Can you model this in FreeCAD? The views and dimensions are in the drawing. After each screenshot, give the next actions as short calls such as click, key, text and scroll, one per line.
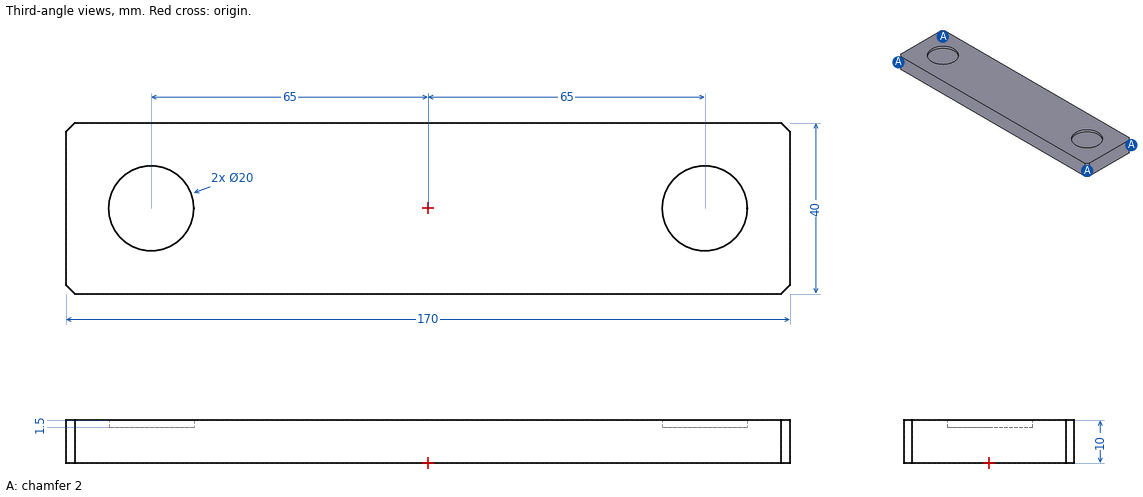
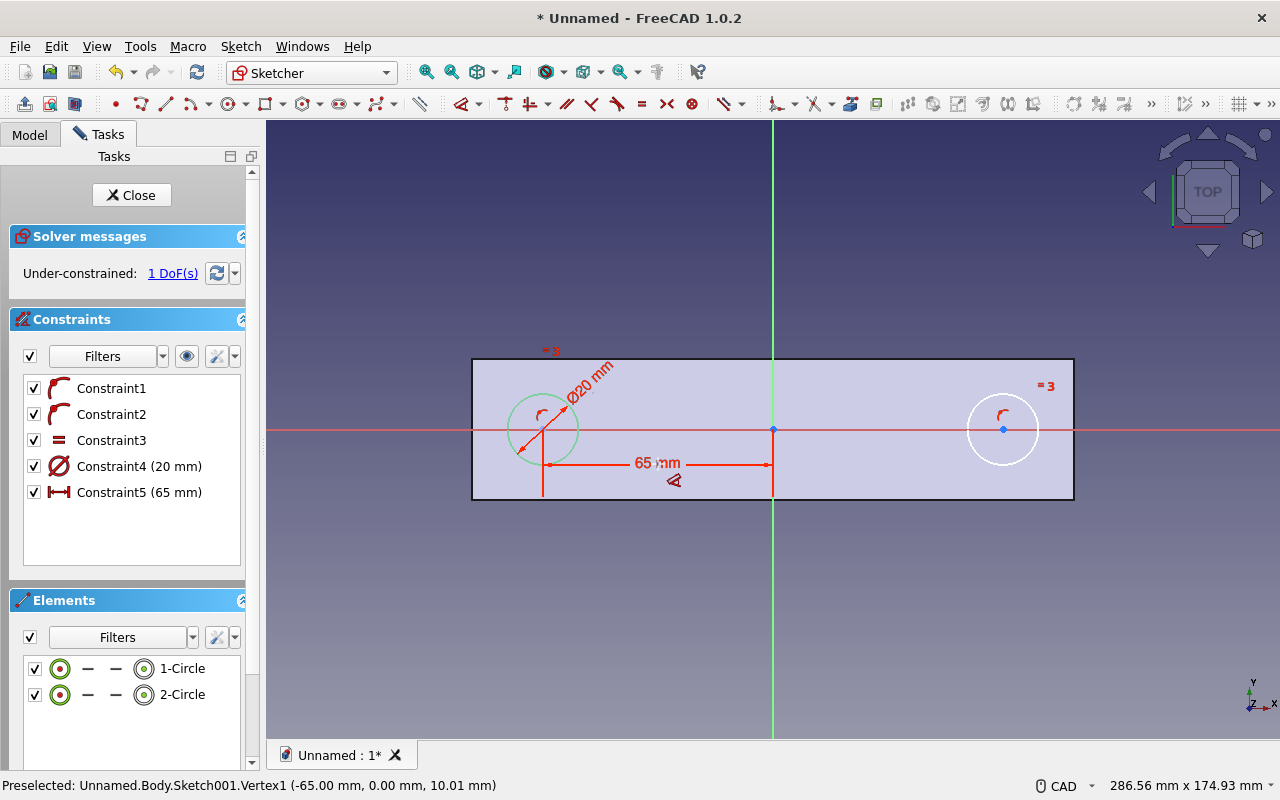
click(1003, 430)
click(888, 464)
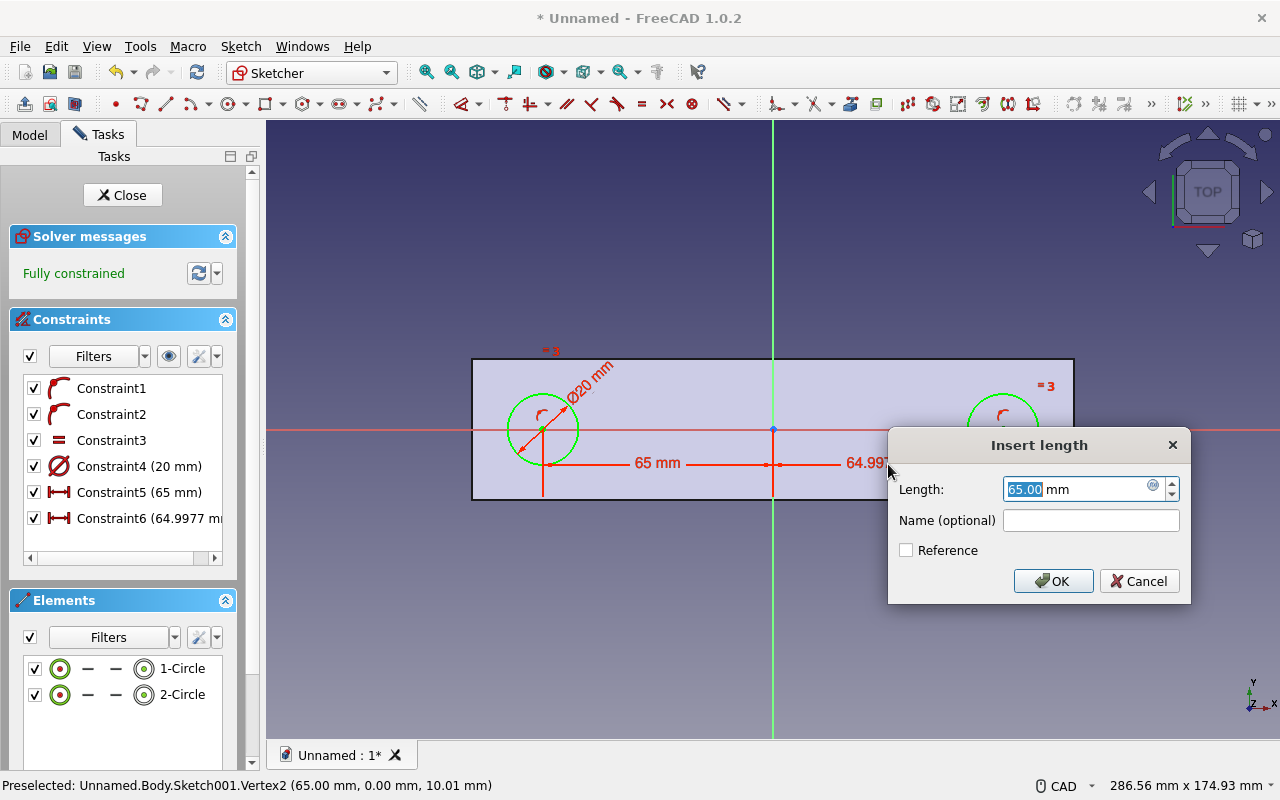
text(65)
key(Return)
key(Escape)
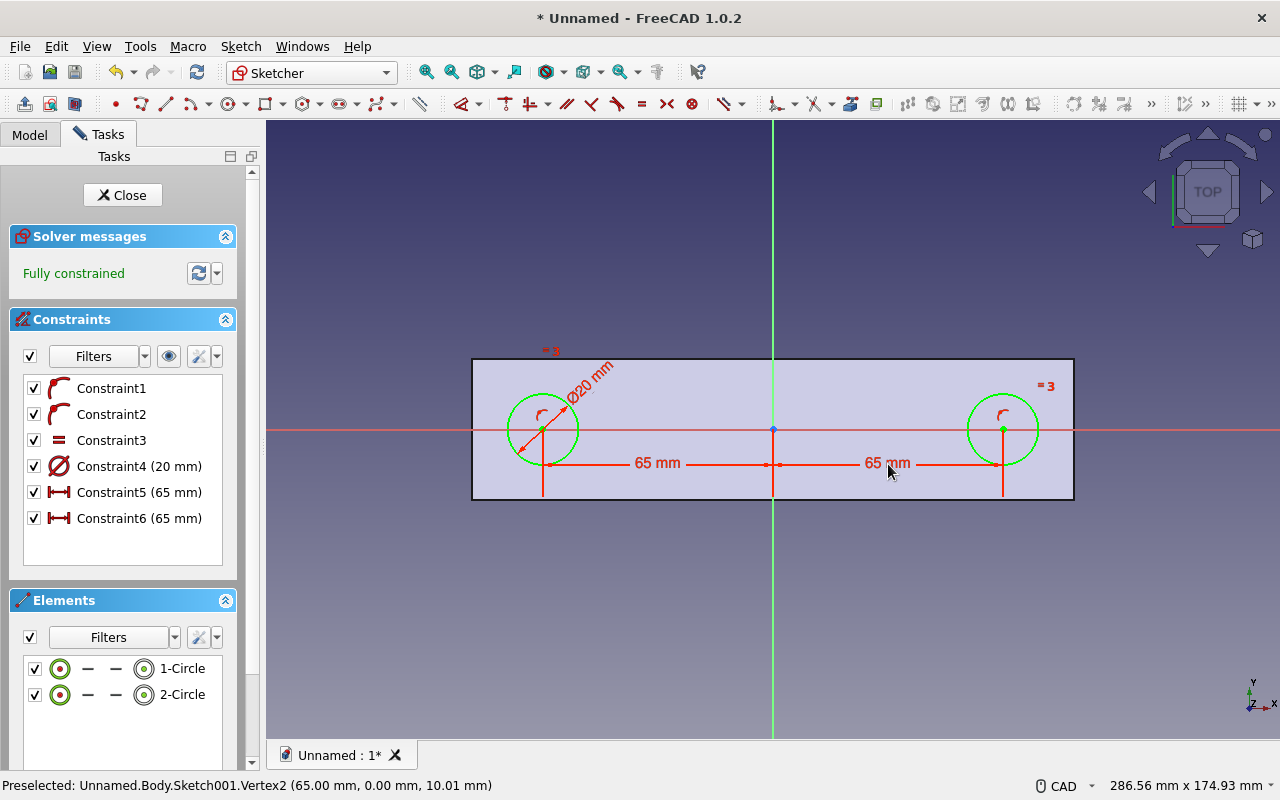
click(123, 195)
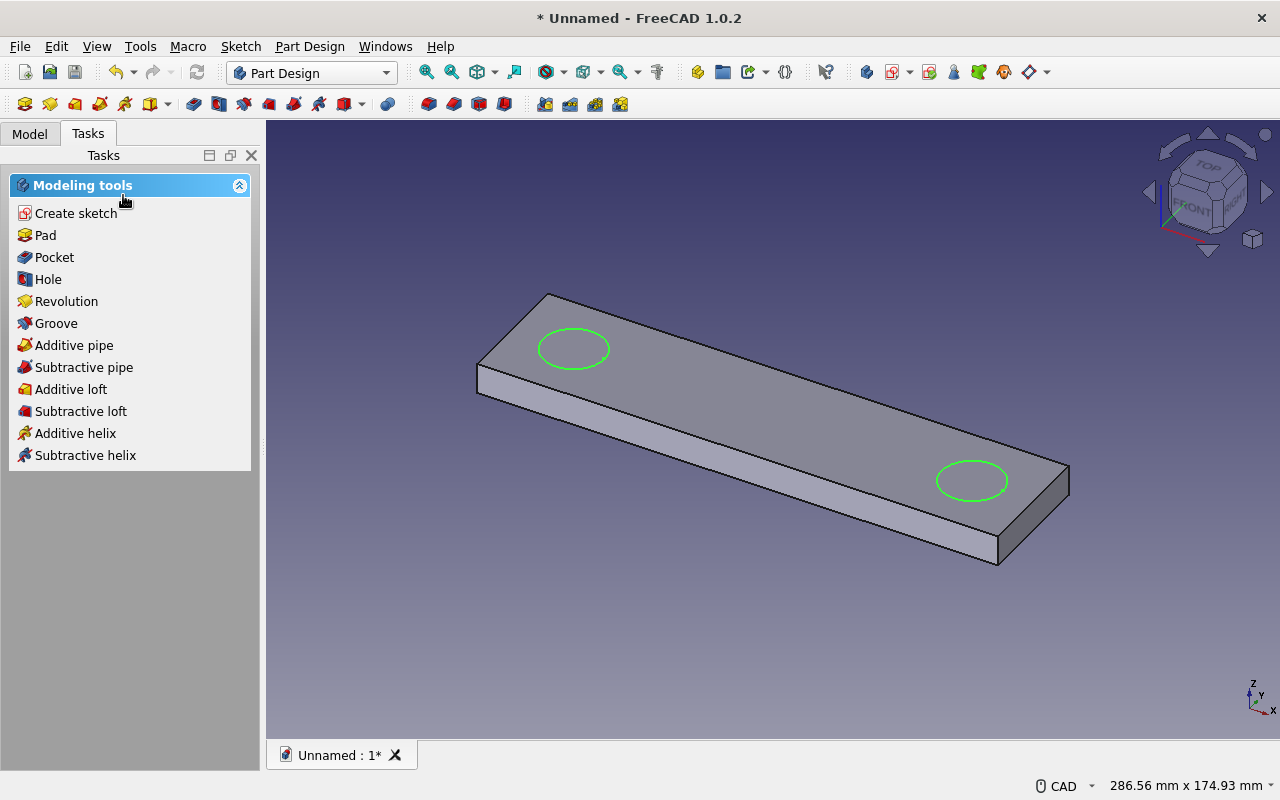
click(194, 104)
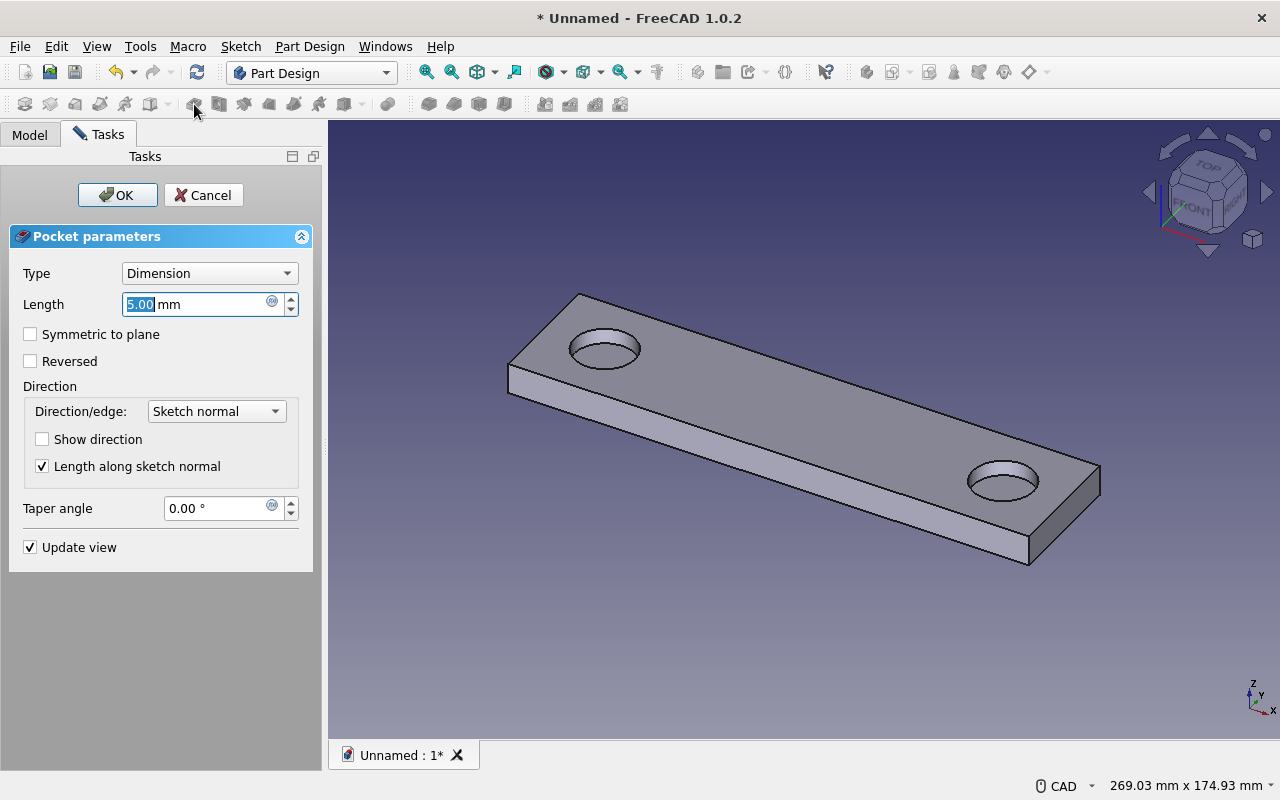
text(1.5)
key(Tab)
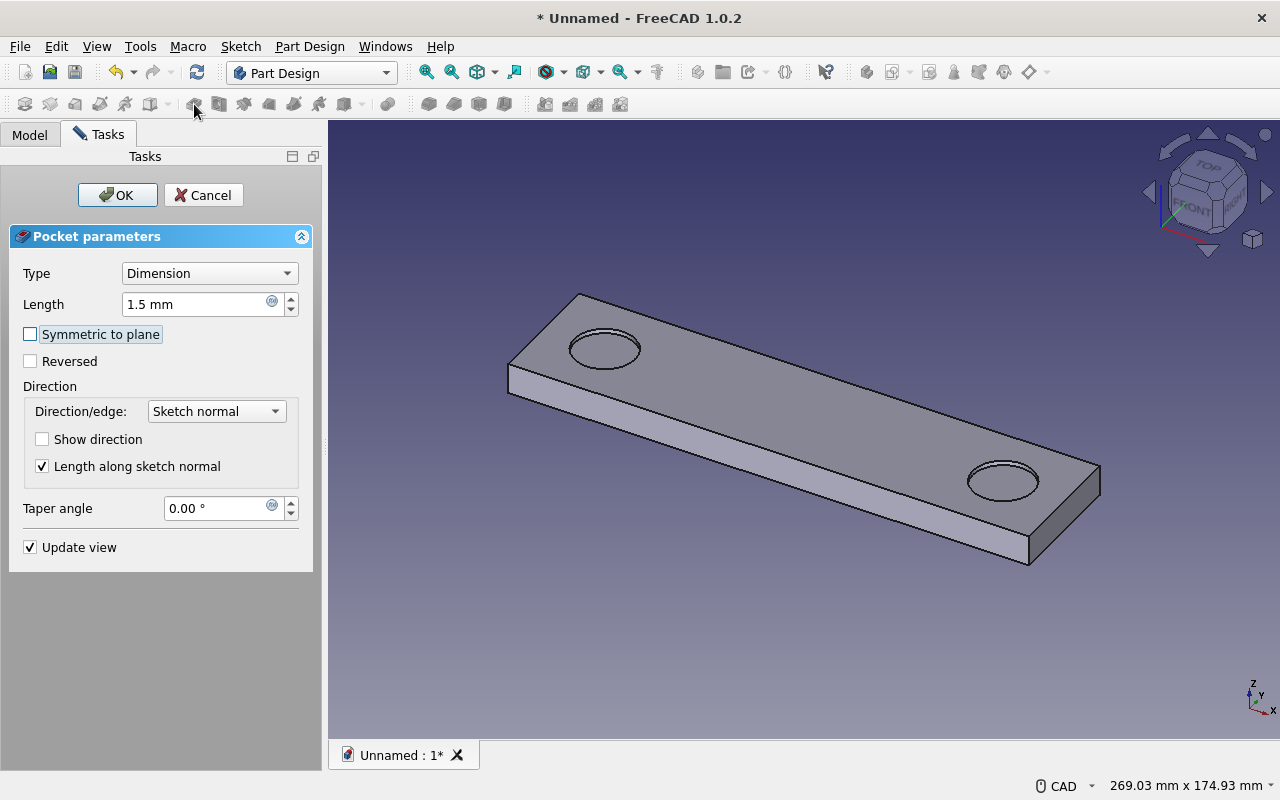
click(118, 195)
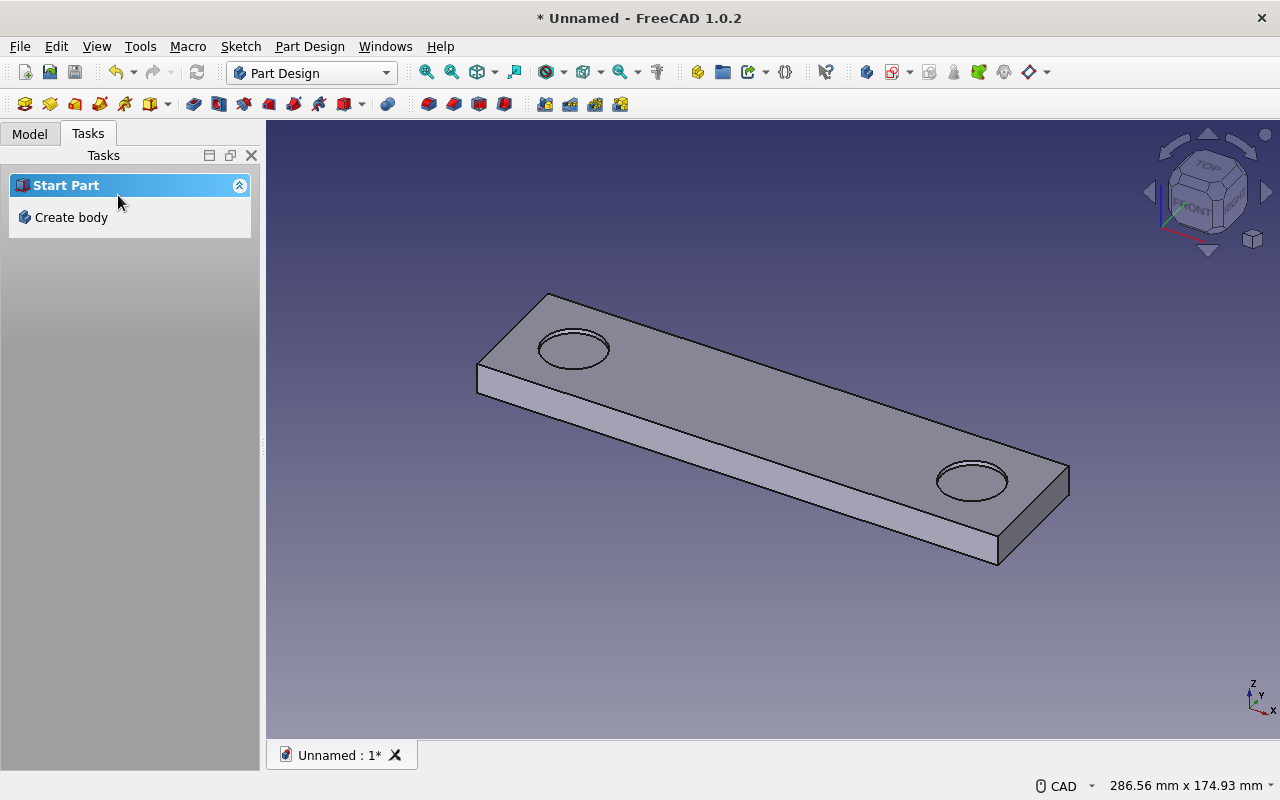
click(998, 550)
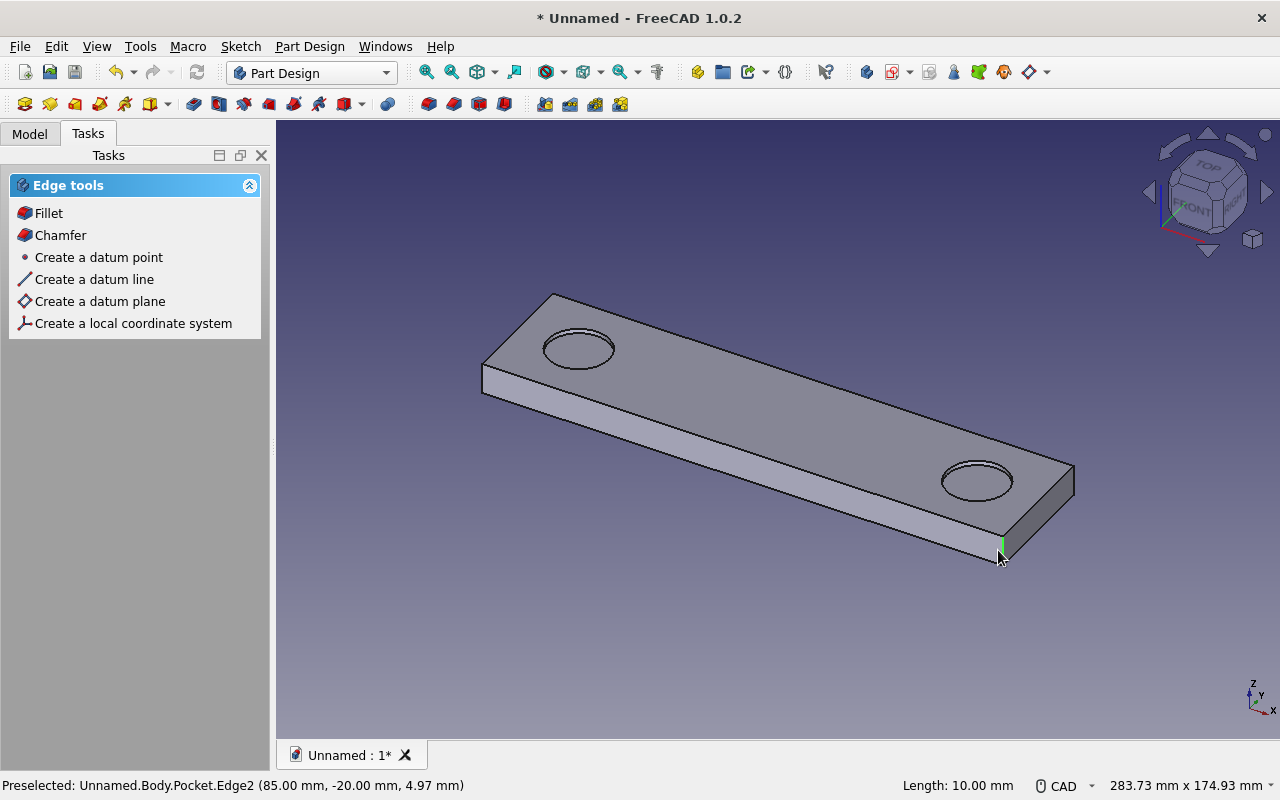
key(0)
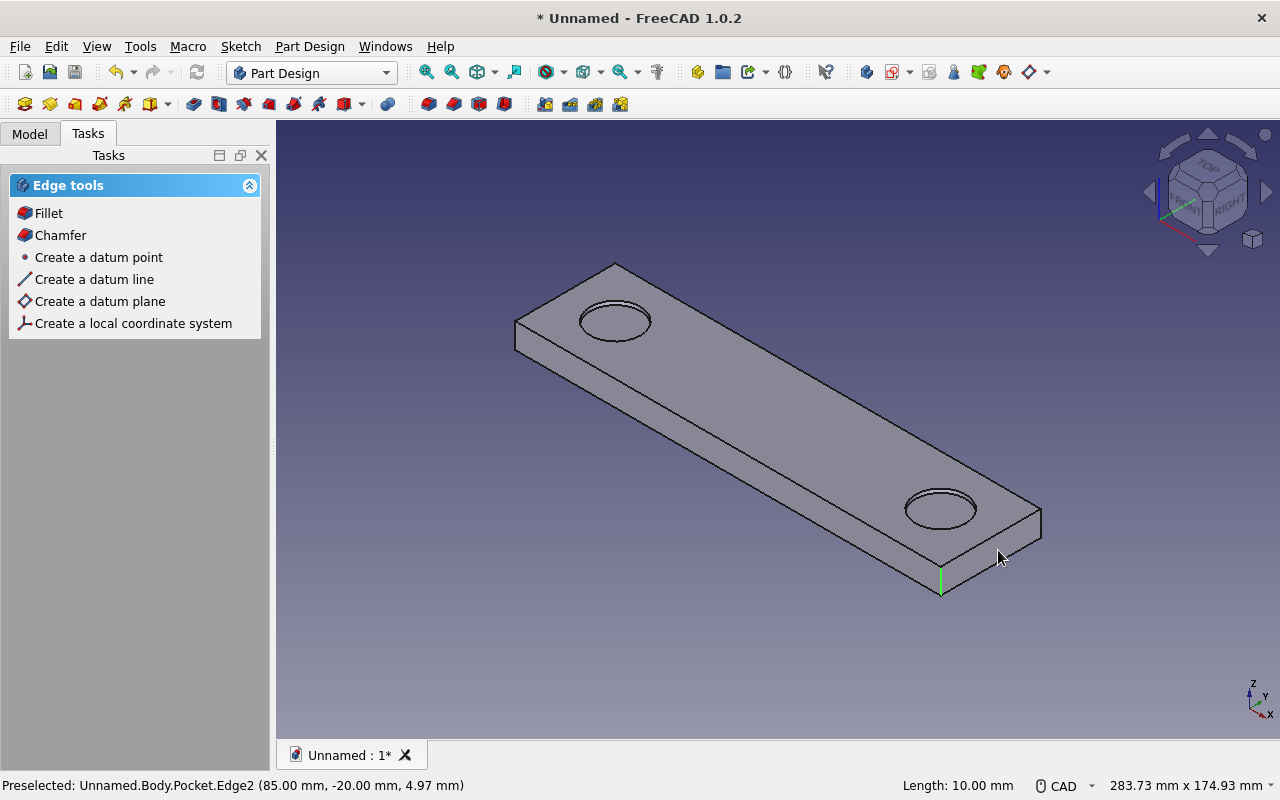
key(2)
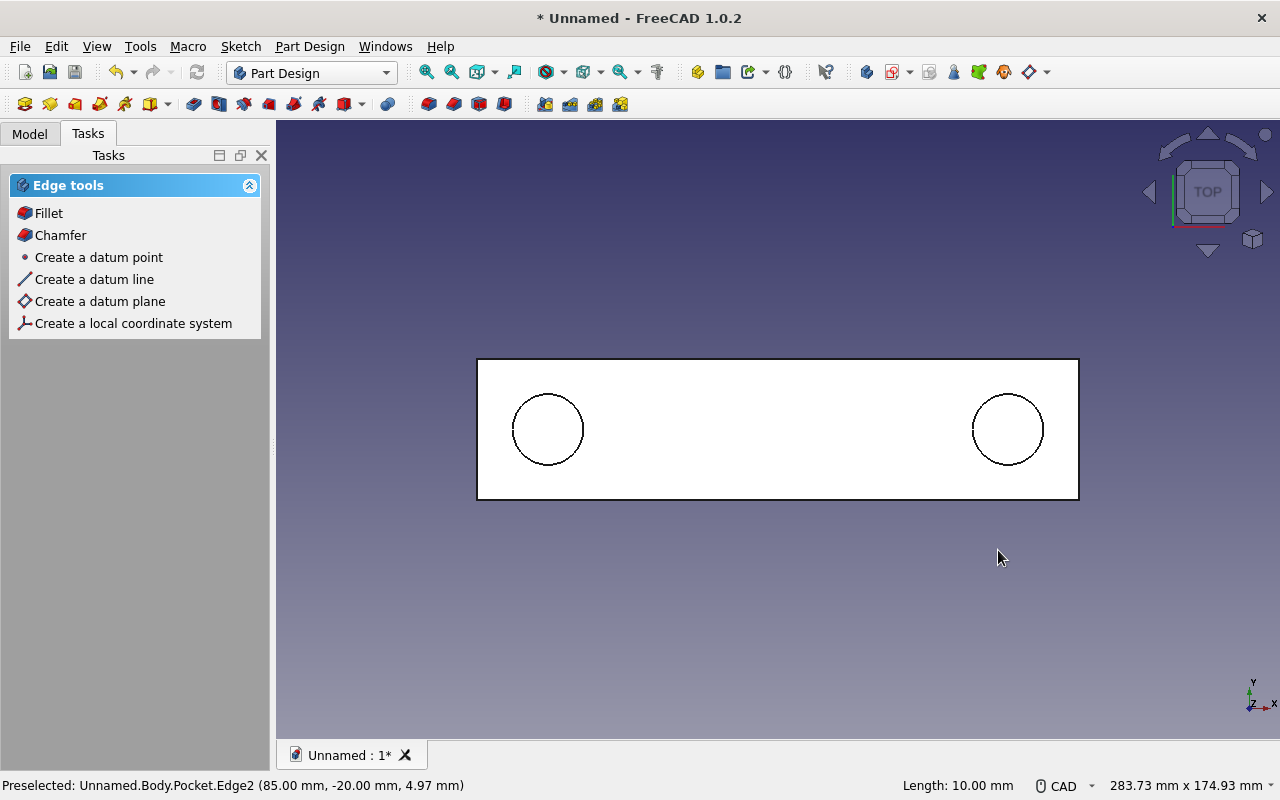
key(1)